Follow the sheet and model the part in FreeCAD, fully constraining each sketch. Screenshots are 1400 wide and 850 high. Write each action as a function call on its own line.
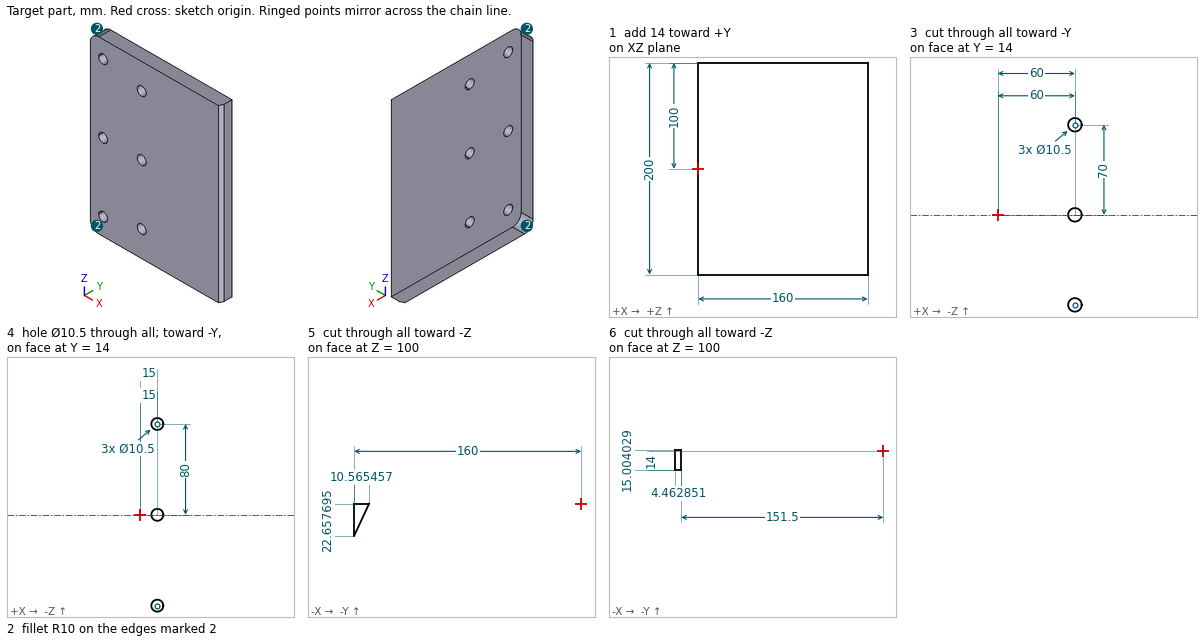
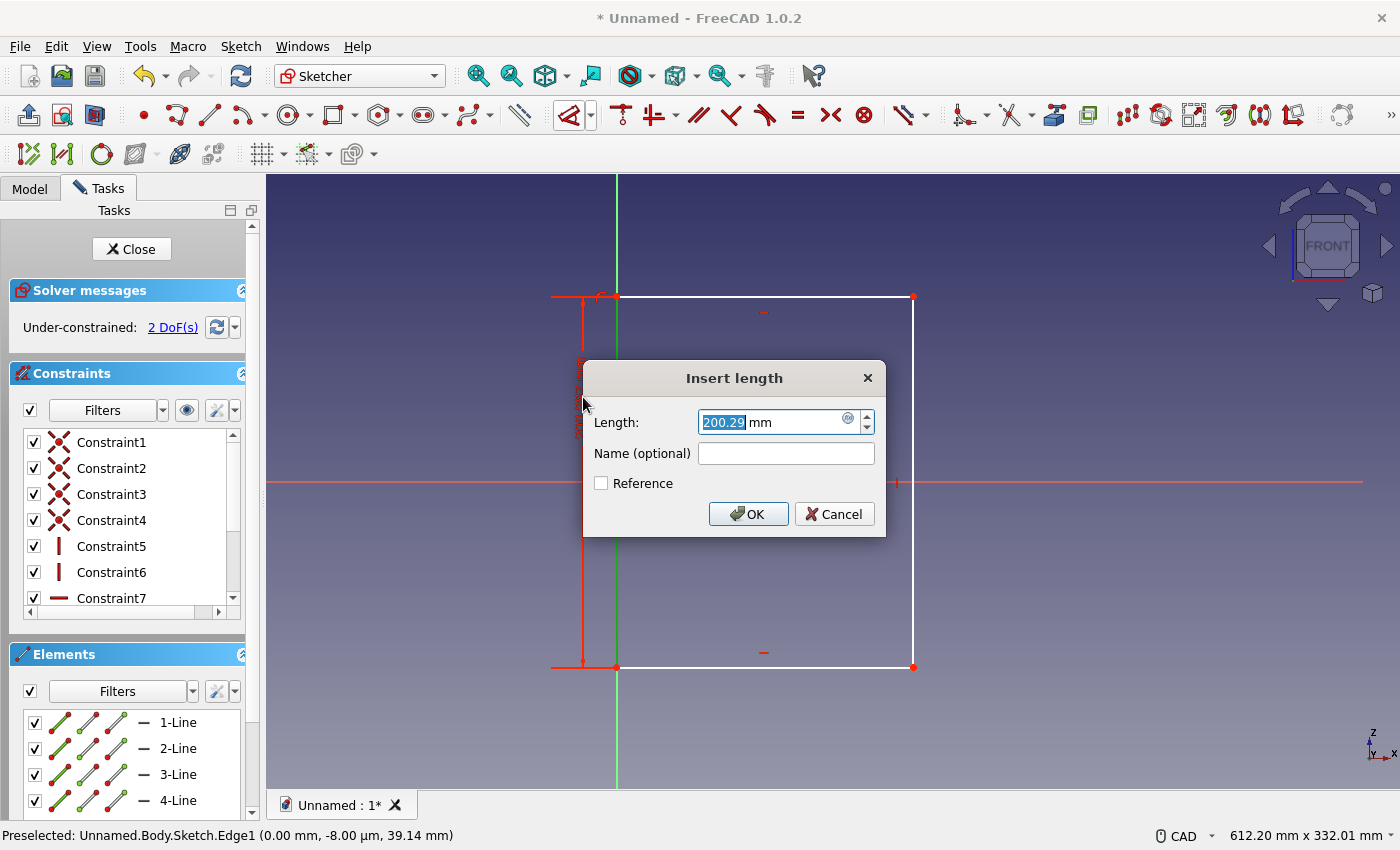
text(200)
key(Return)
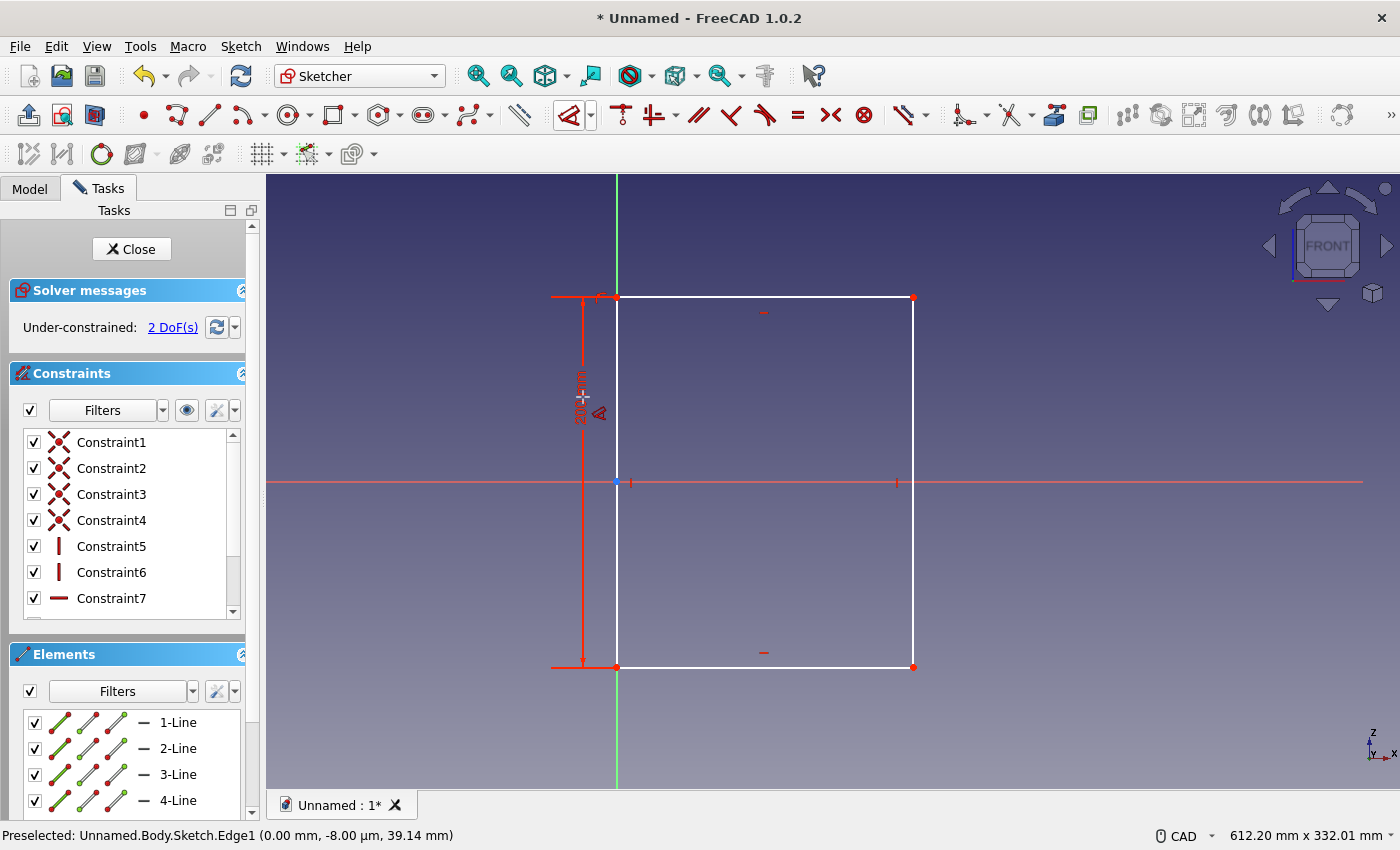
click(705, 668)
click(765, 702)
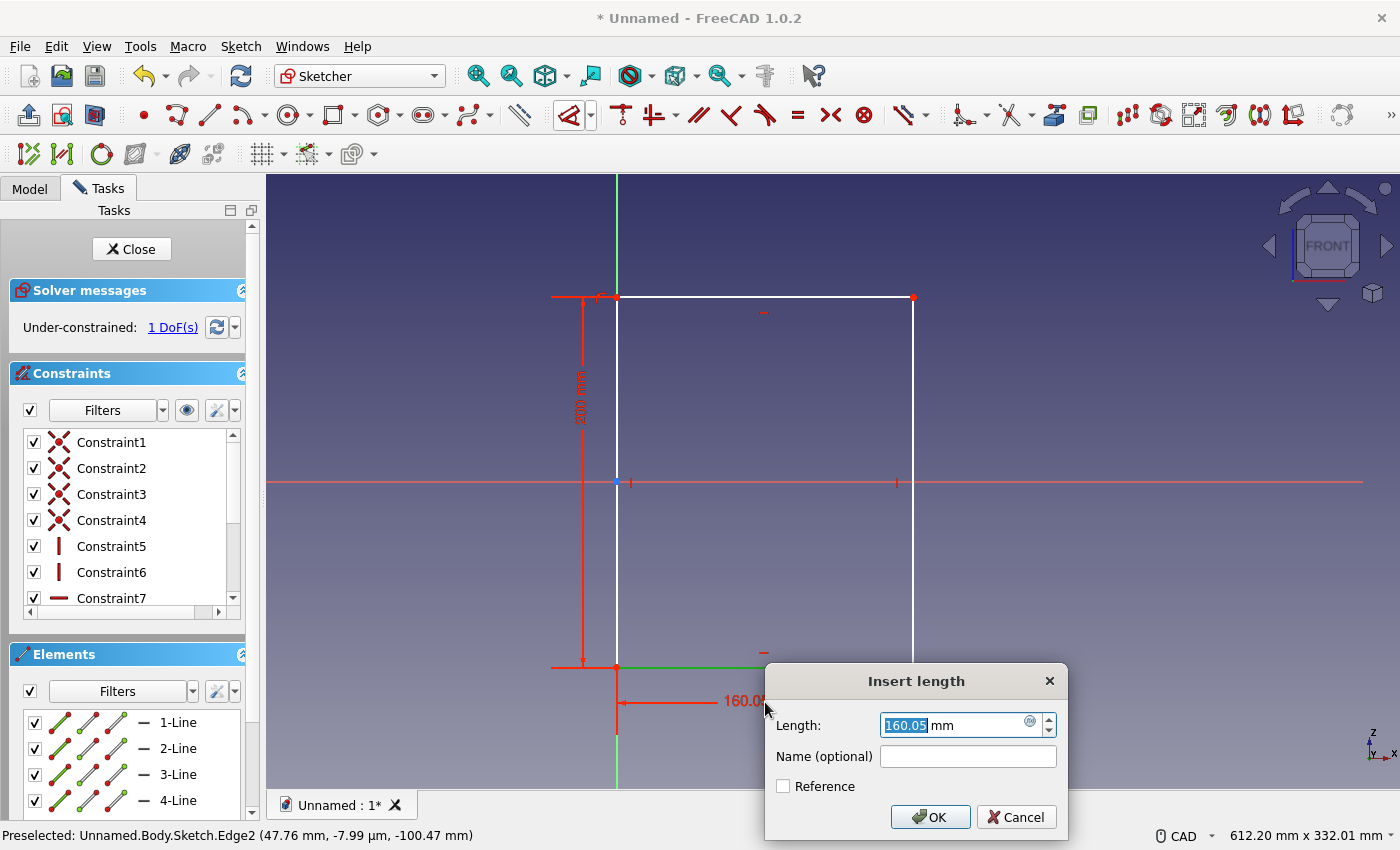
text(160)
key(Return)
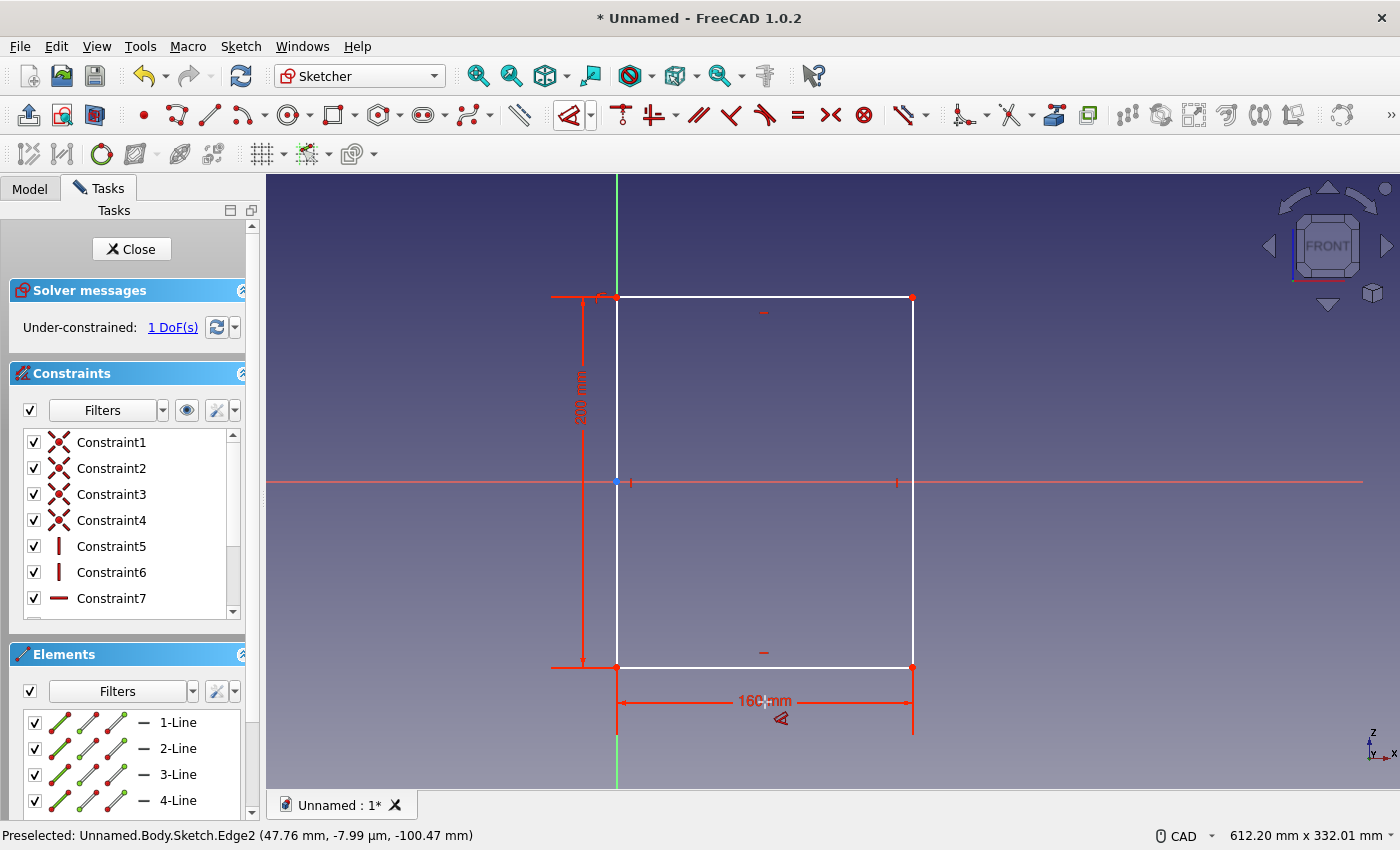
click(617, 297)
click(583, 347)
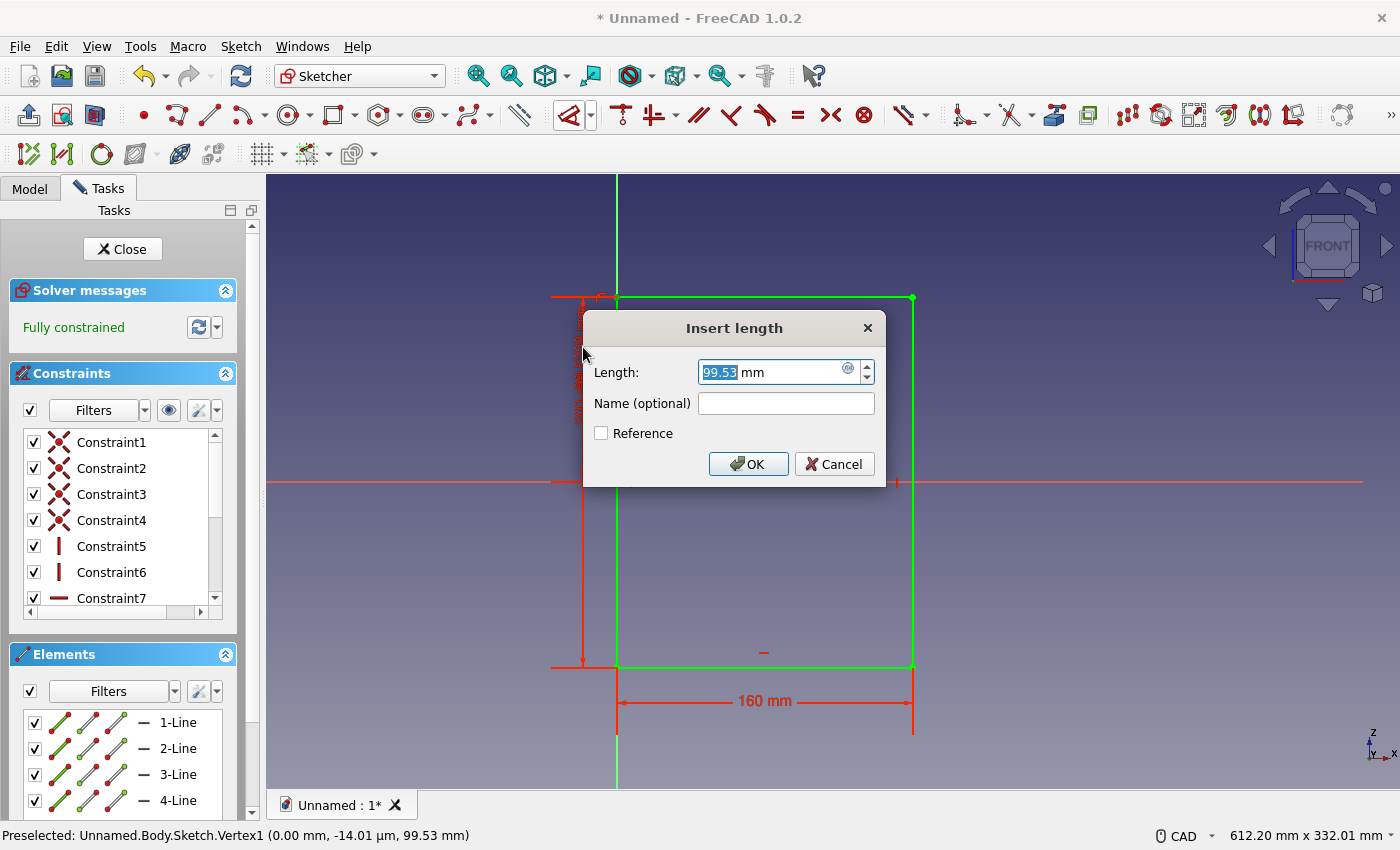
text(100)
key(Return)
key(Escape)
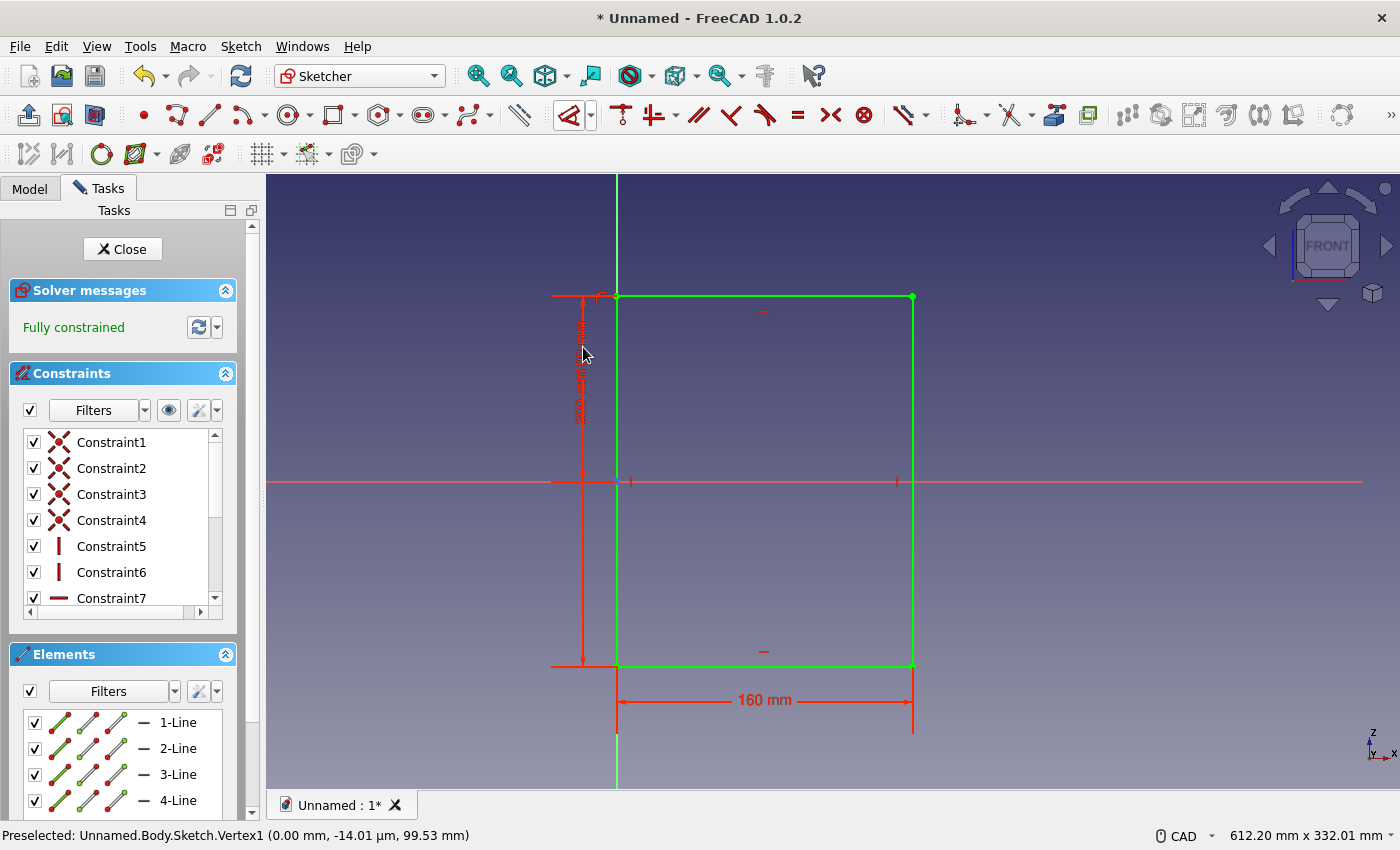
click(123, 249)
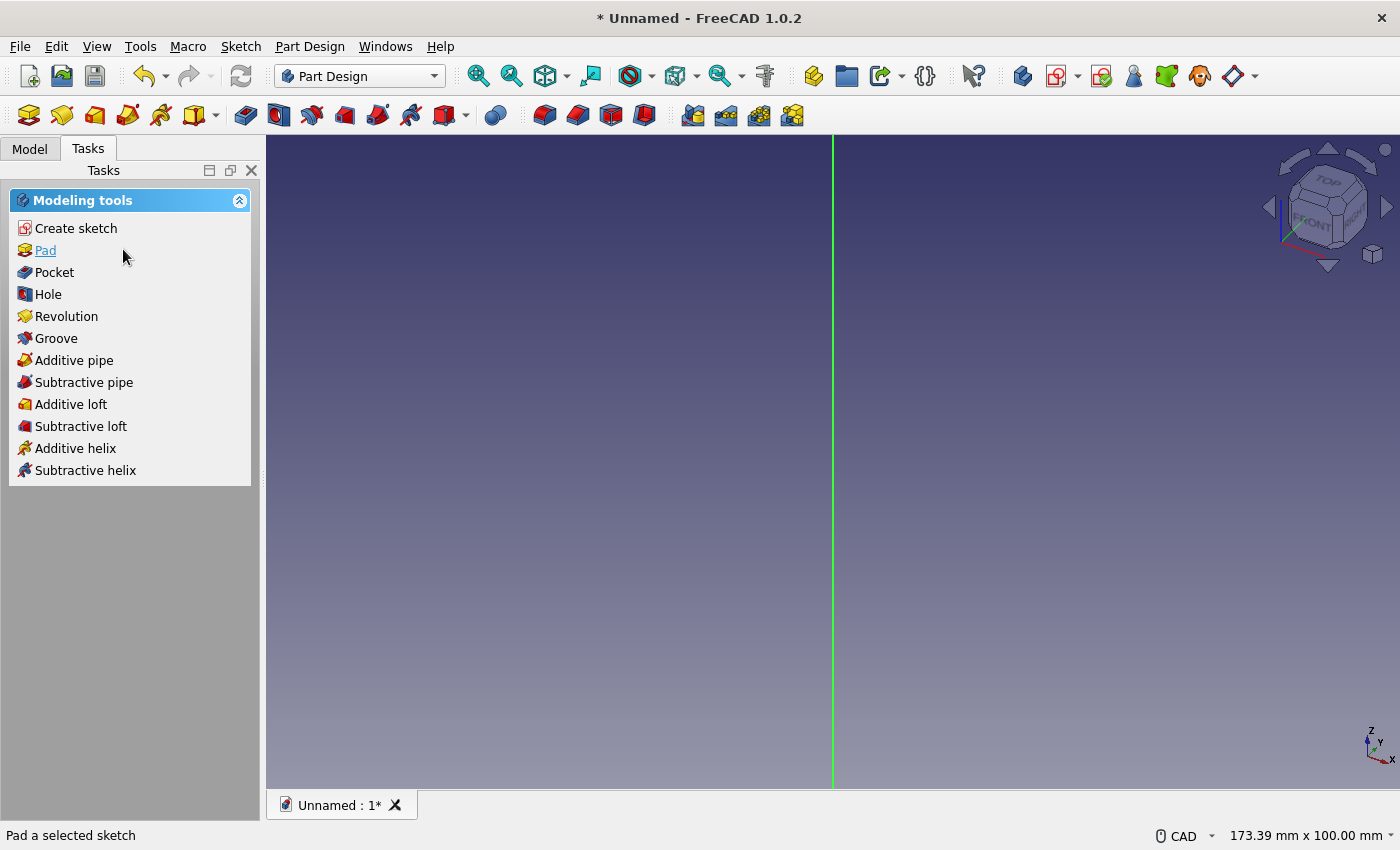
click(29, 116)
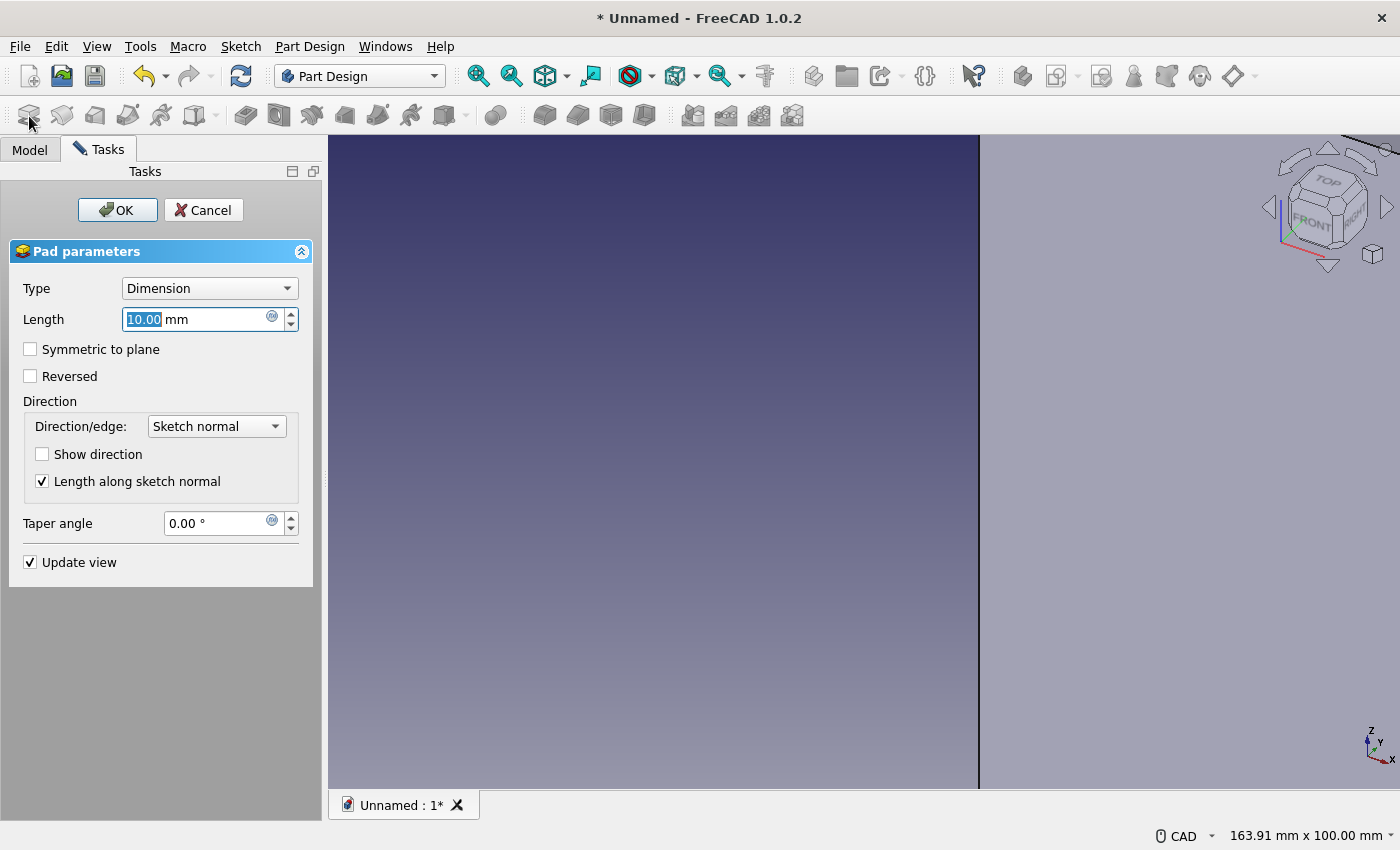
text(14)
key(Tab)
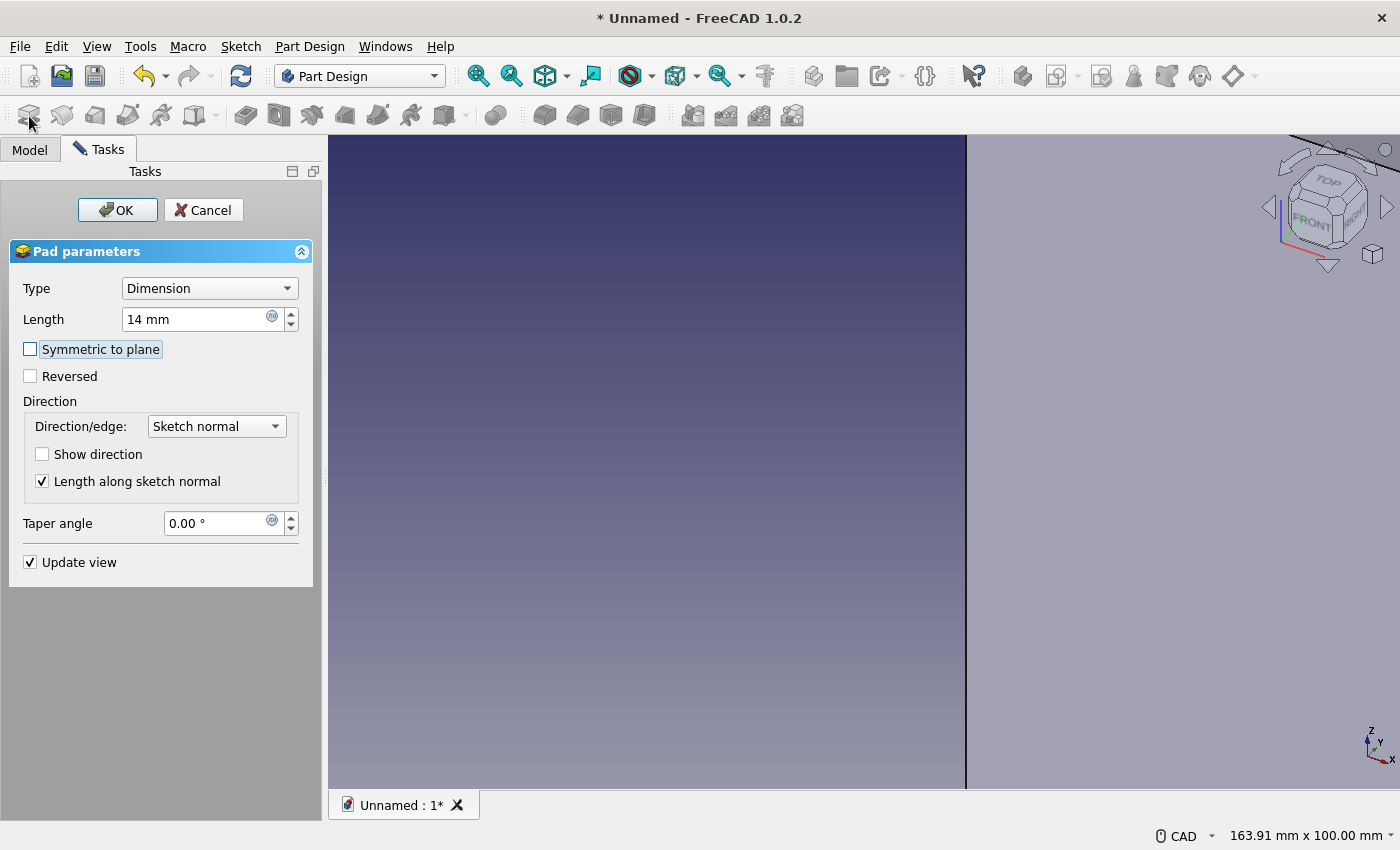
click(31, 376)